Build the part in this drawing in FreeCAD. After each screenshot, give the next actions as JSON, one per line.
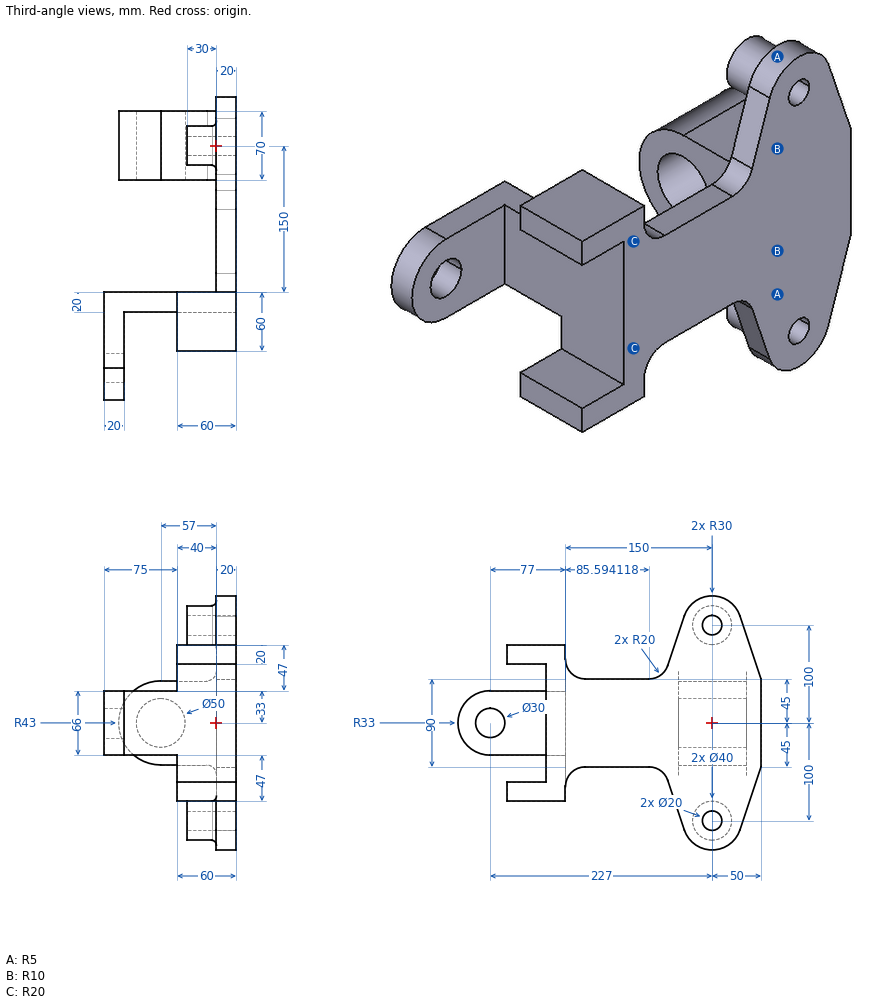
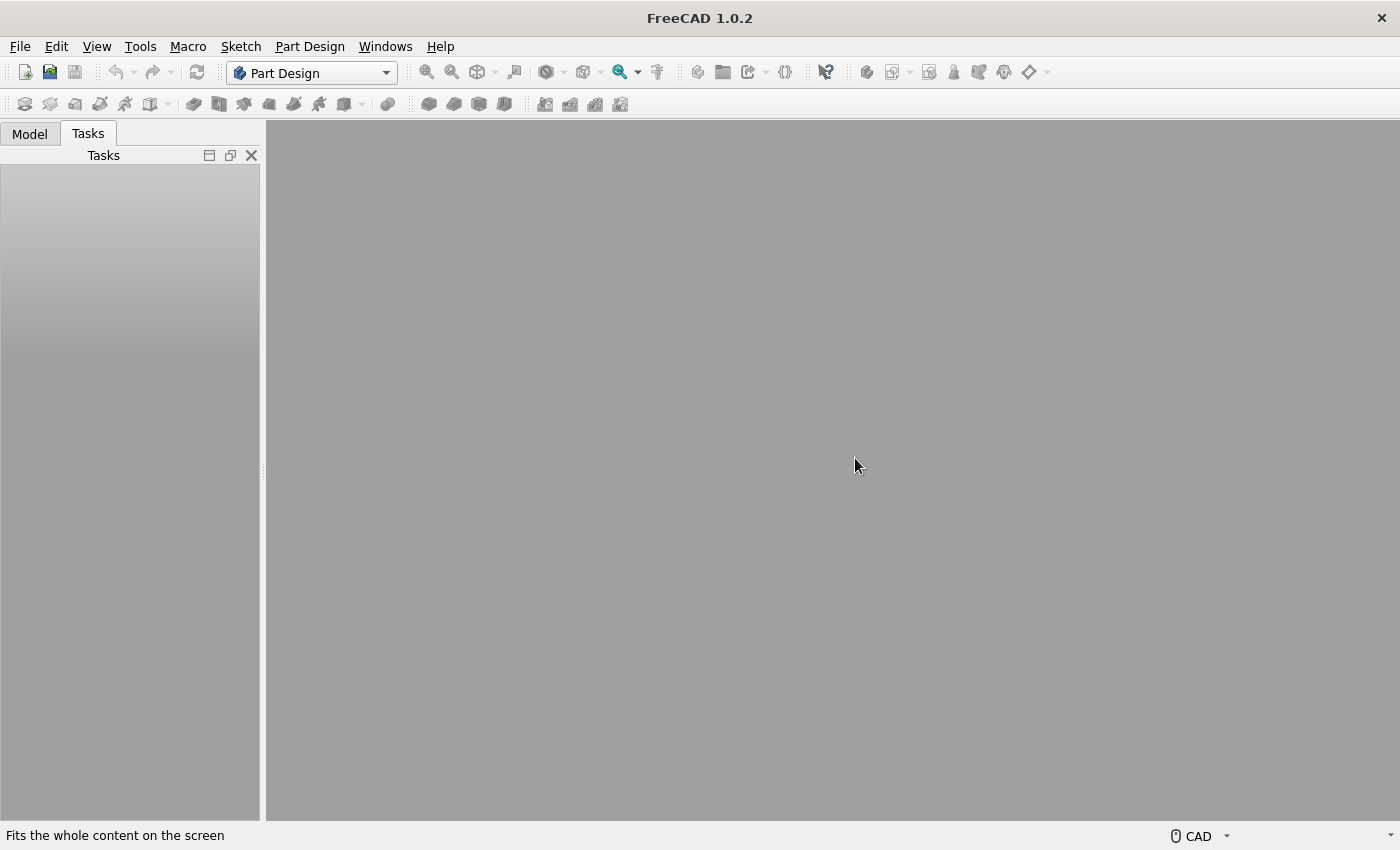
{"action": "key", "text": "ctrl+n"}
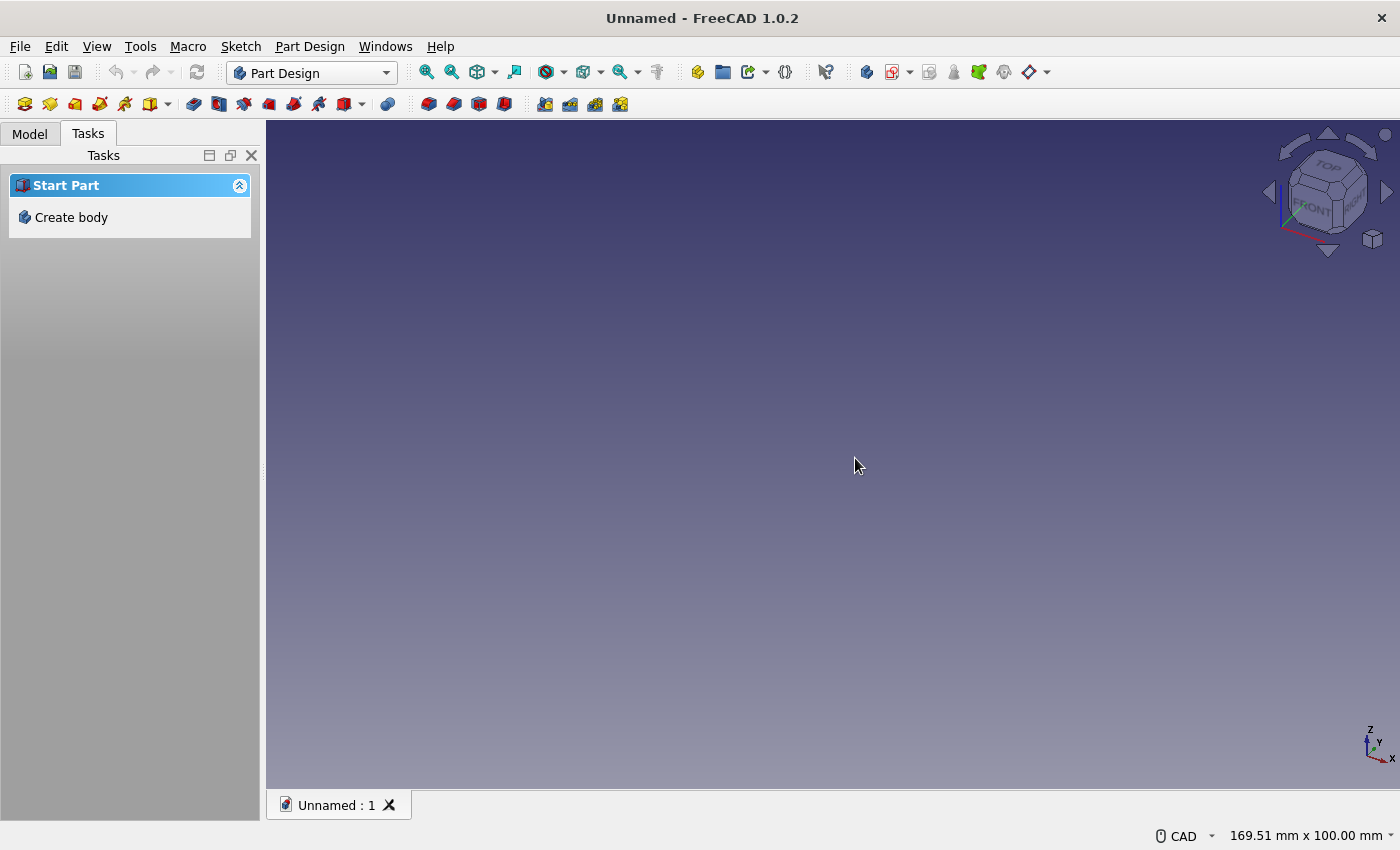
{"action": "left_click", "coordinate": [892, 72]}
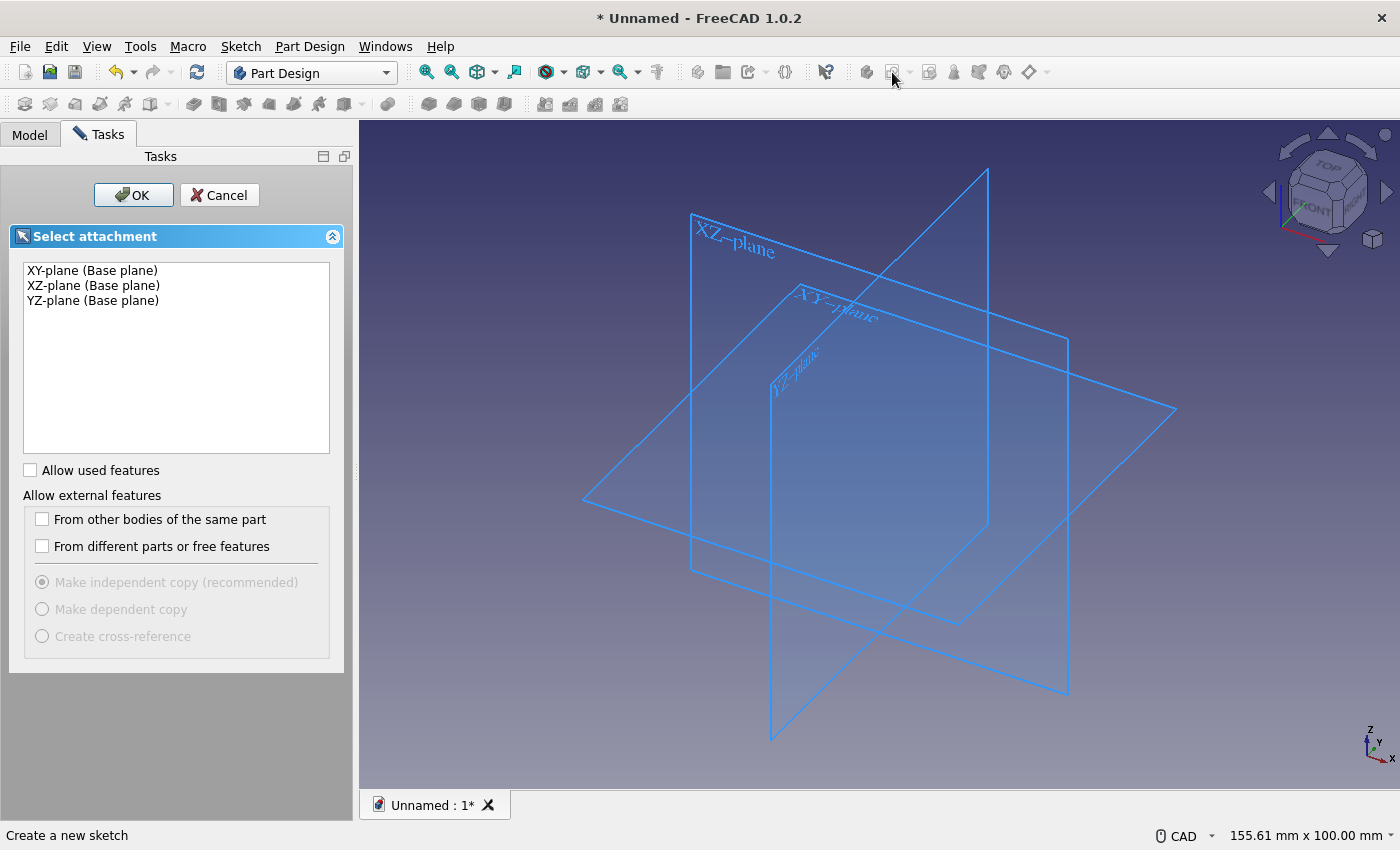
{"action": "left_click", "coordinate": [84, 300]}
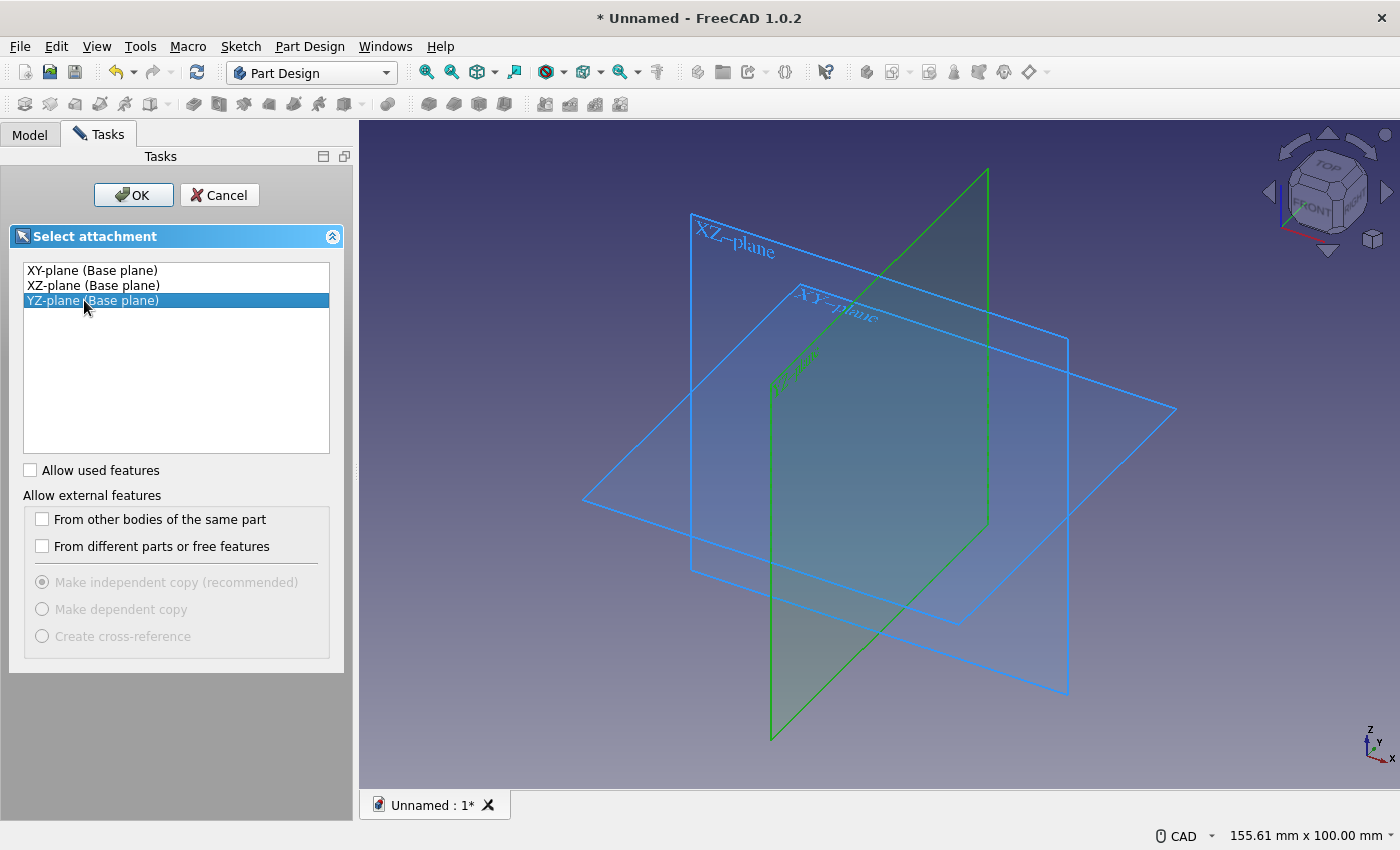
{"action": "left_click", "coordinate": [134, 195]}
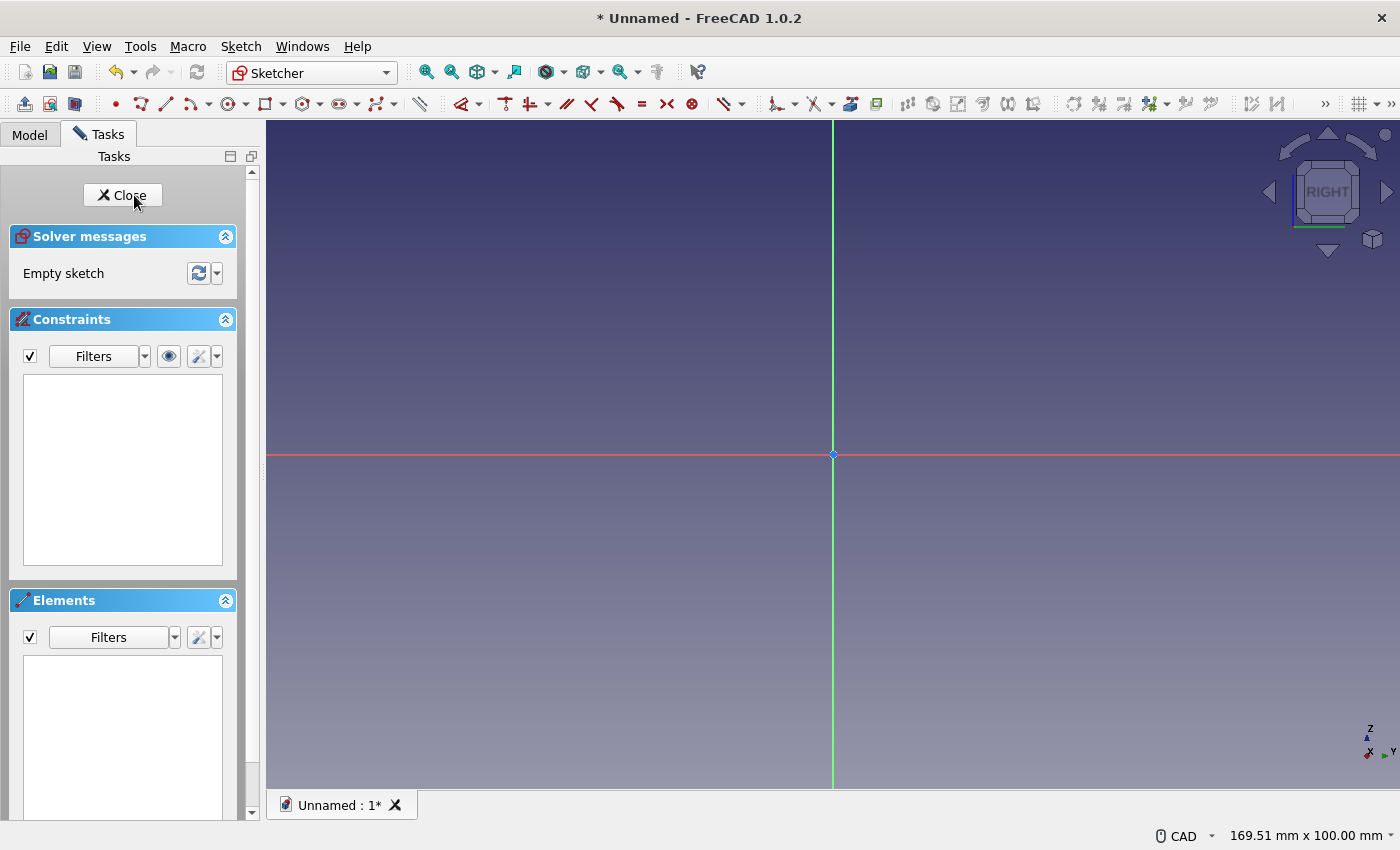
{"action": "scroll", "coordinate": [852, 454], "scroll_direction": "down", "scroll_amount": 7}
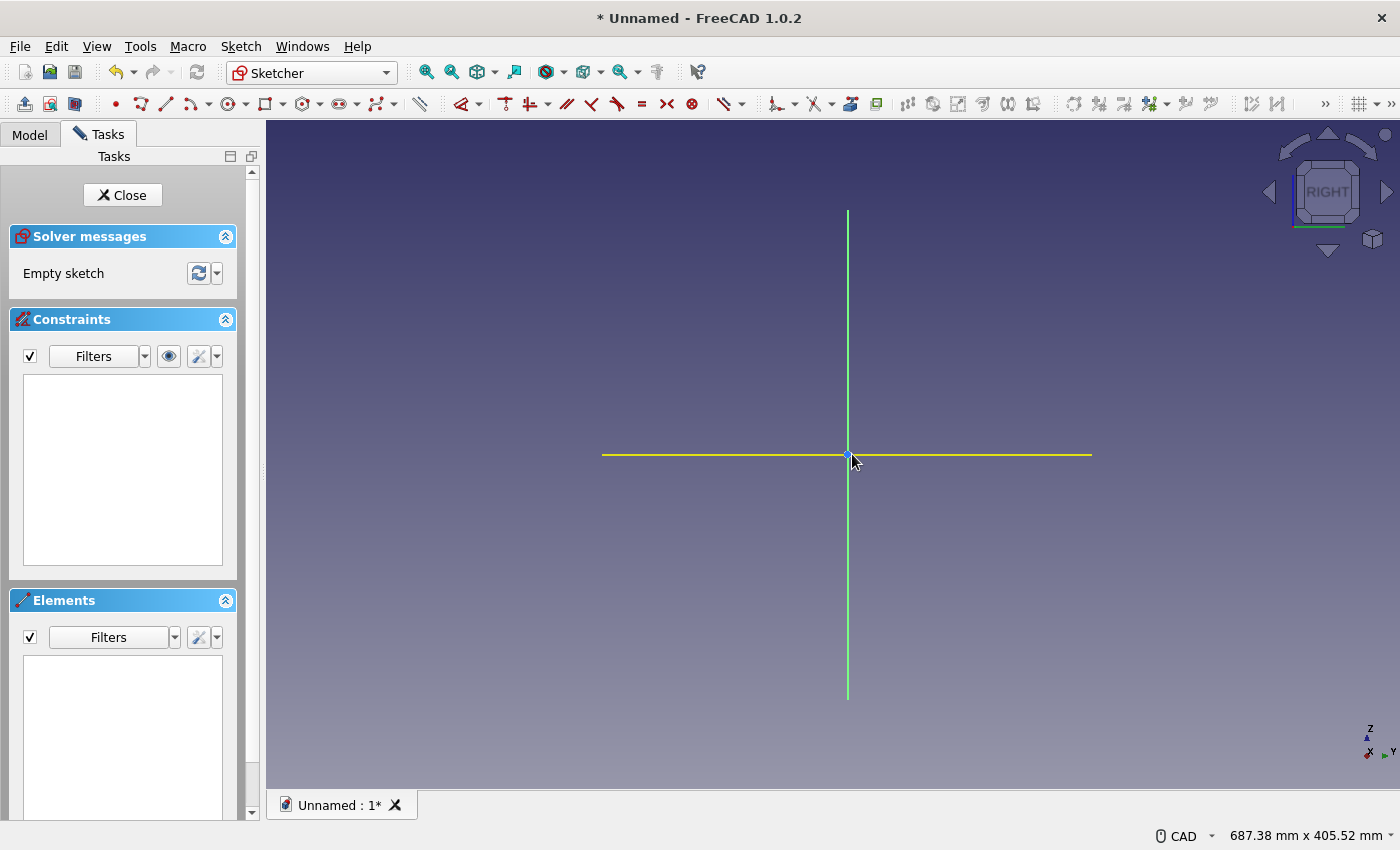
{"action": "left_click", "coordinate": [166, 104]}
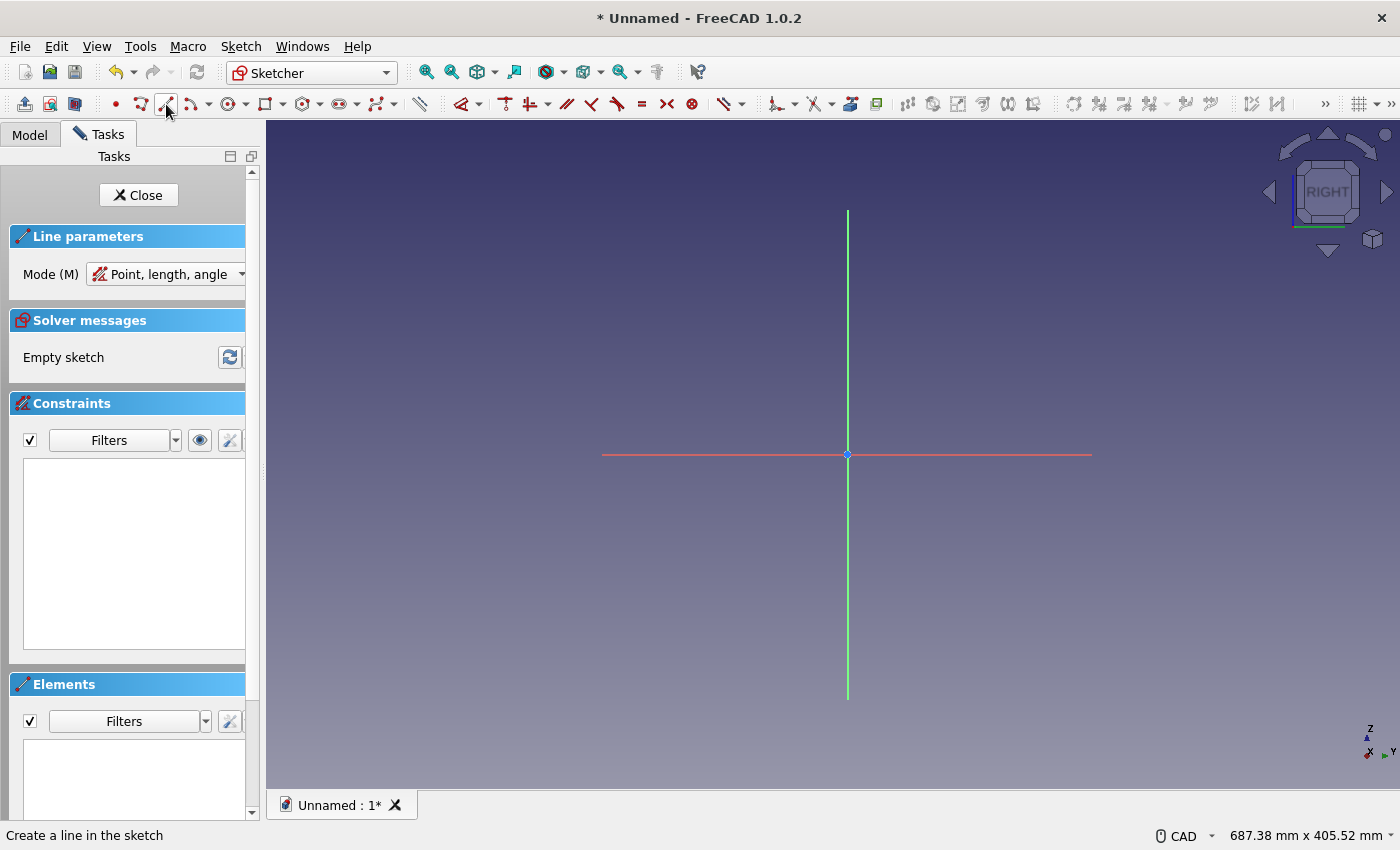
{"action": "left_click", "coordinate": [801, 274]}
{"action": "left_click", "coordinate": [773, 358]}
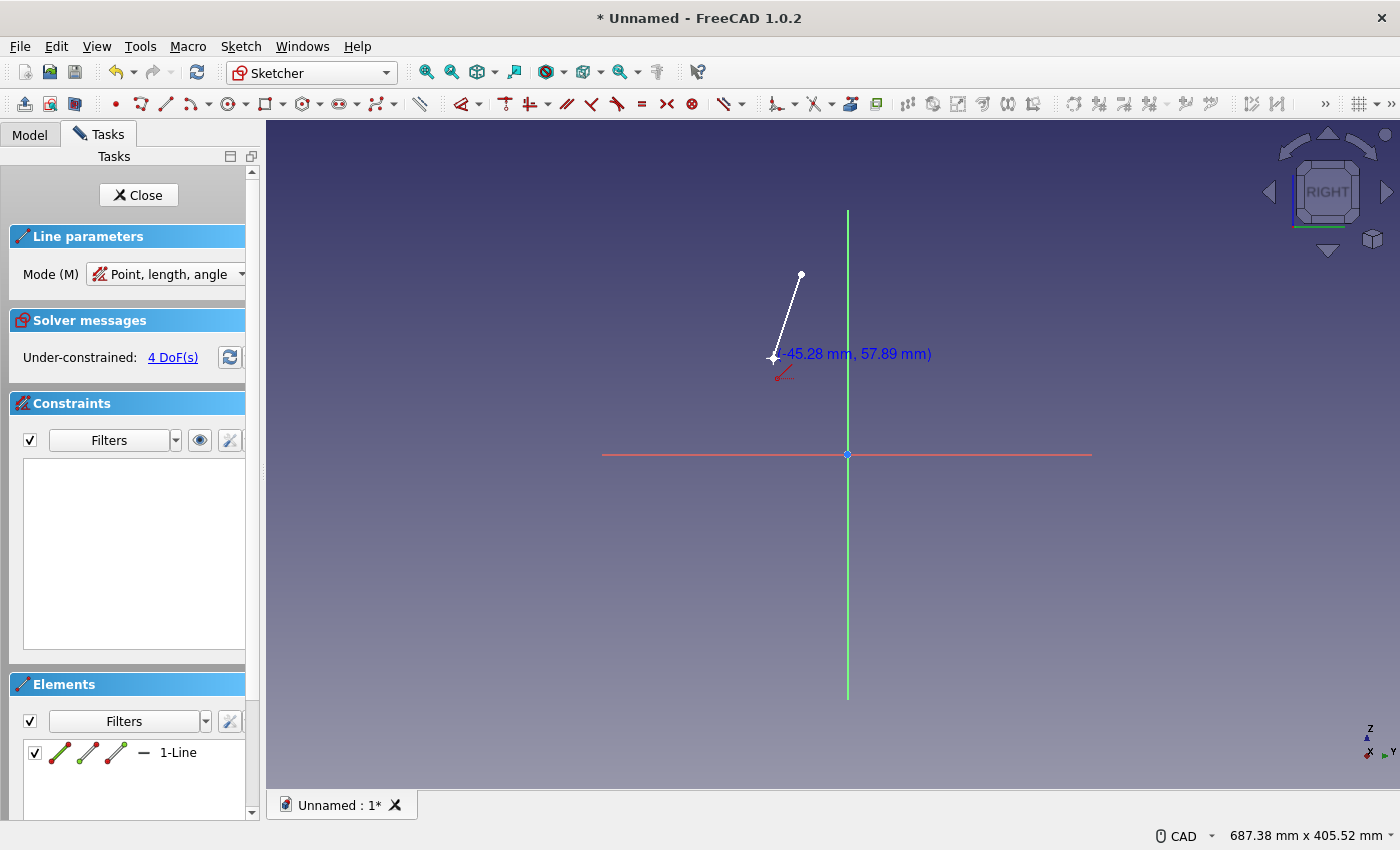
{"action": "left_click", "coordinate": [141, 104]}